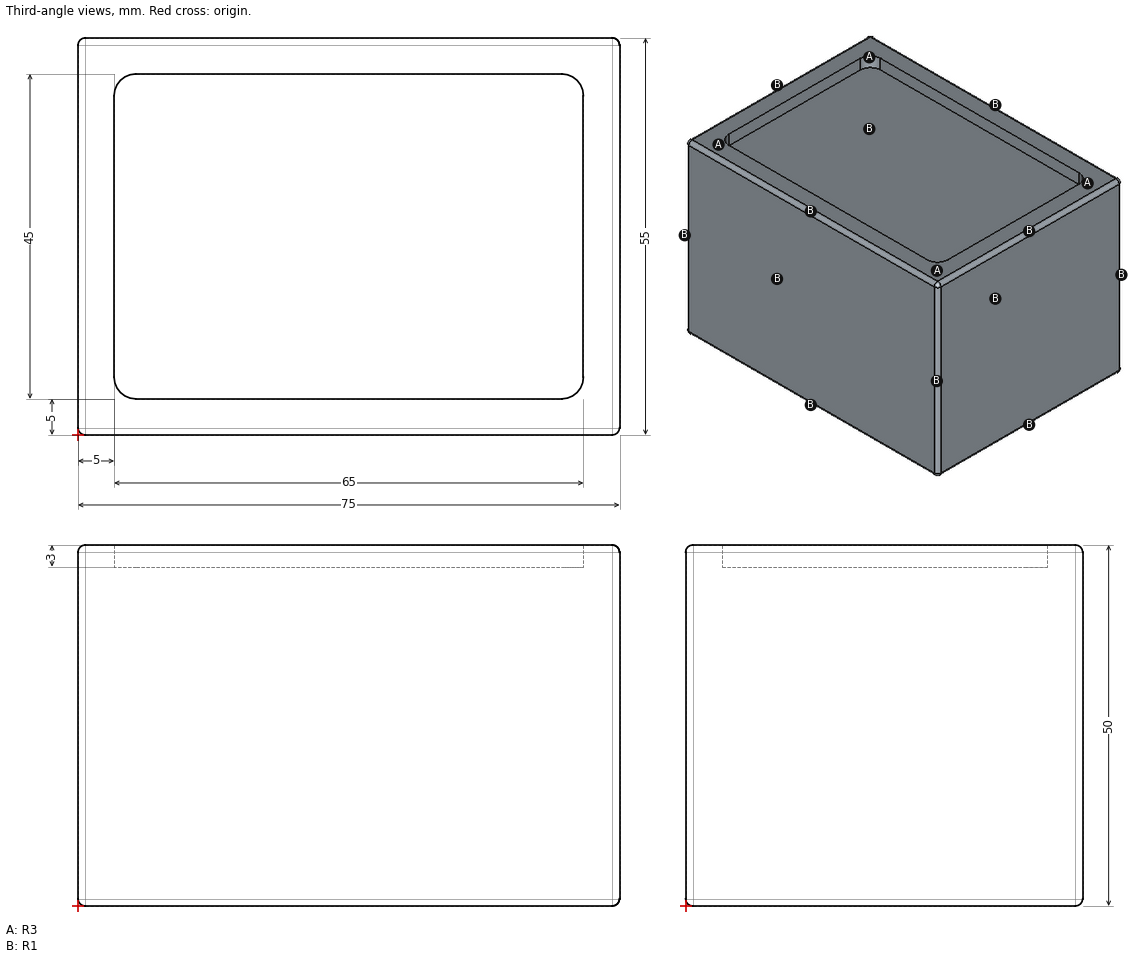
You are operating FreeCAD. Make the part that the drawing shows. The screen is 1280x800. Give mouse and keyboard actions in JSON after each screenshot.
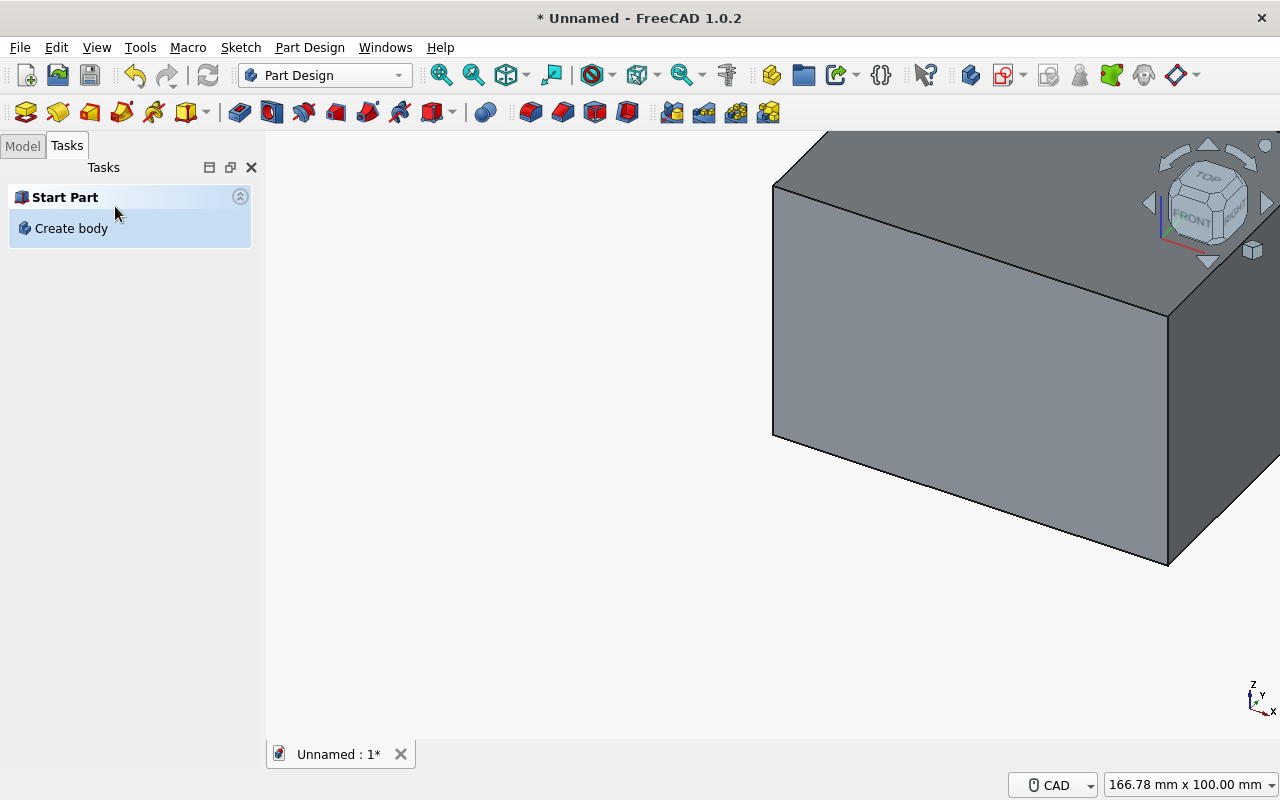
{"action": "left_click", "coordinate": [442, 76]}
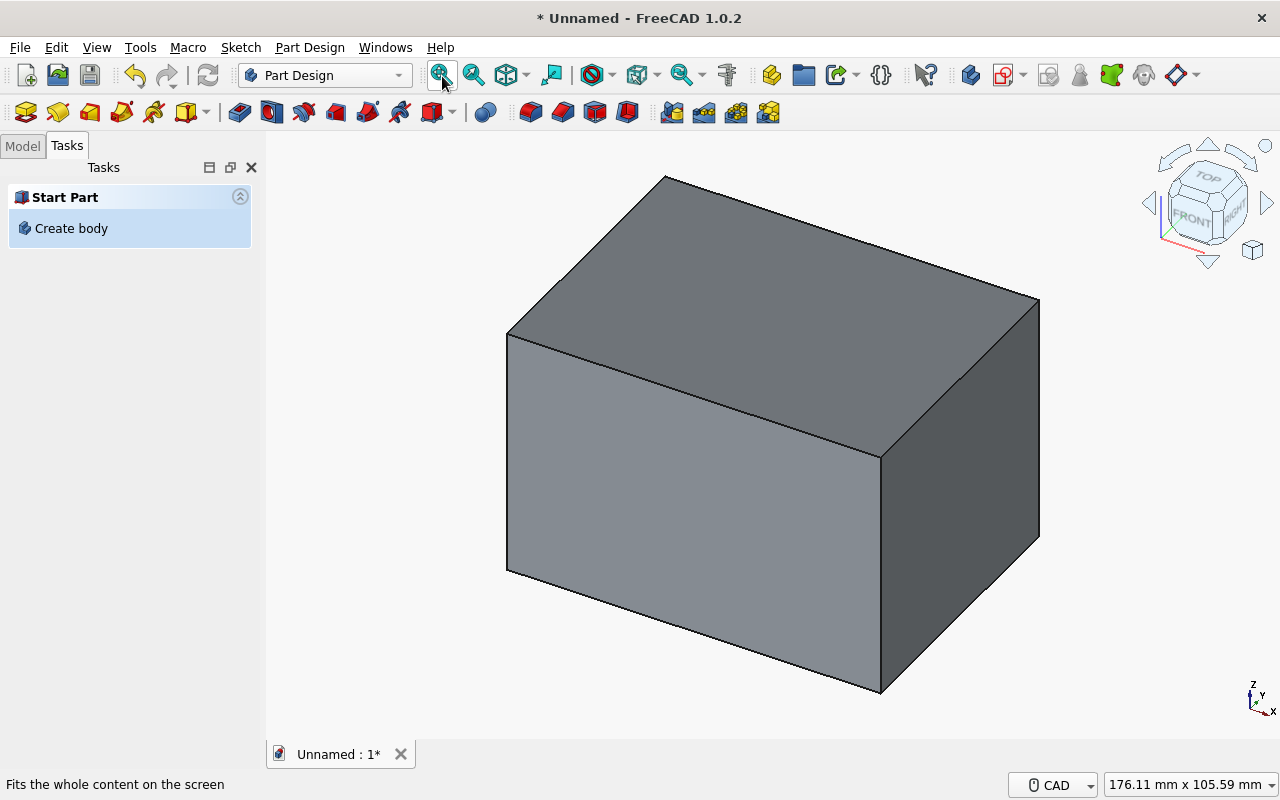
{"action": "left_click", "coordinate": [773, 316]}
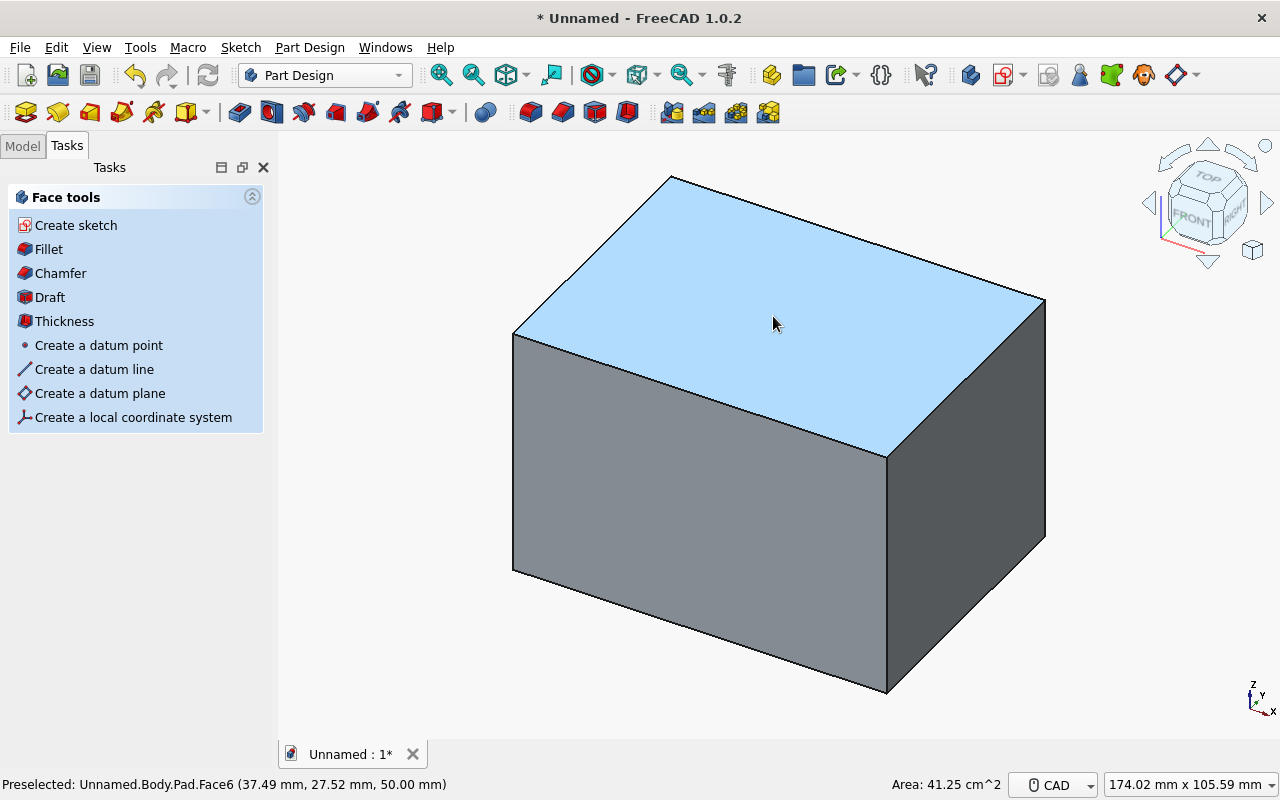
{"action": "left_click", "coordinate": [1004, 76]}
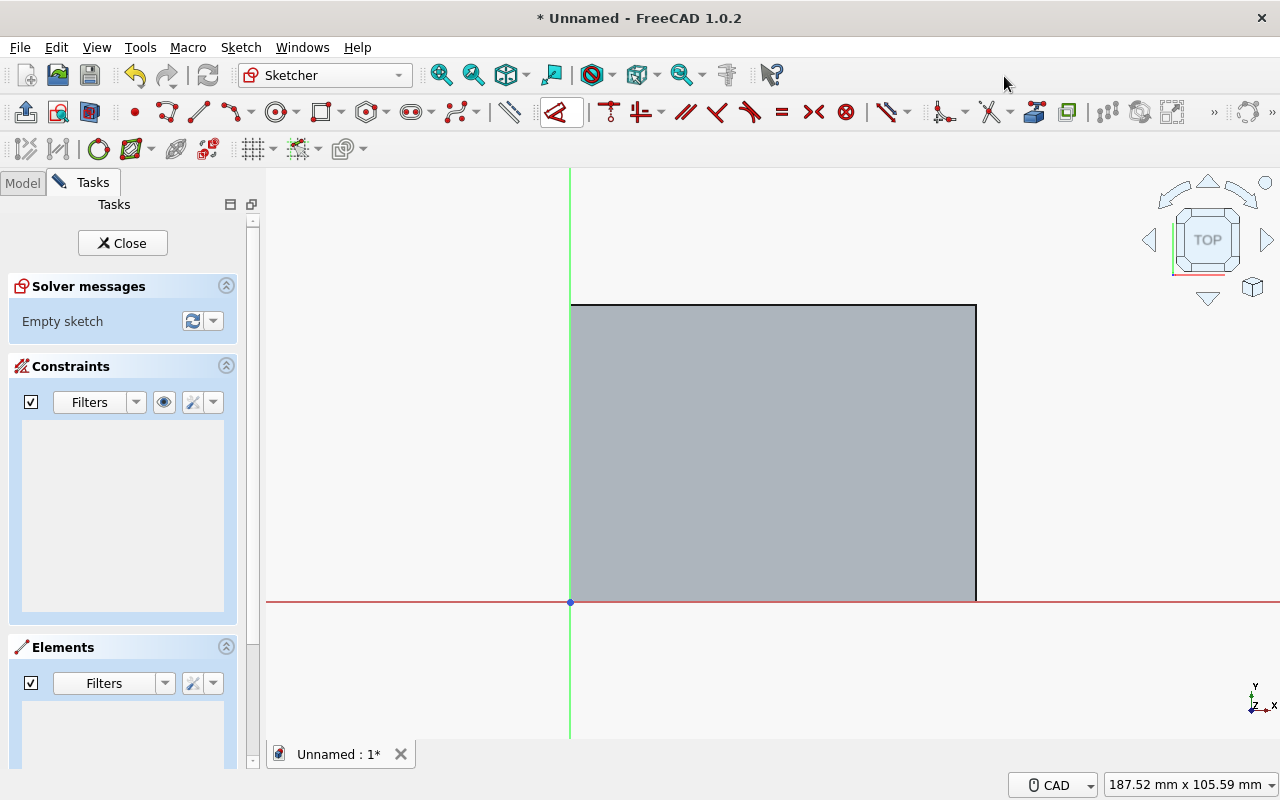
{"action": "left_click", "coordinate": [322, 112]}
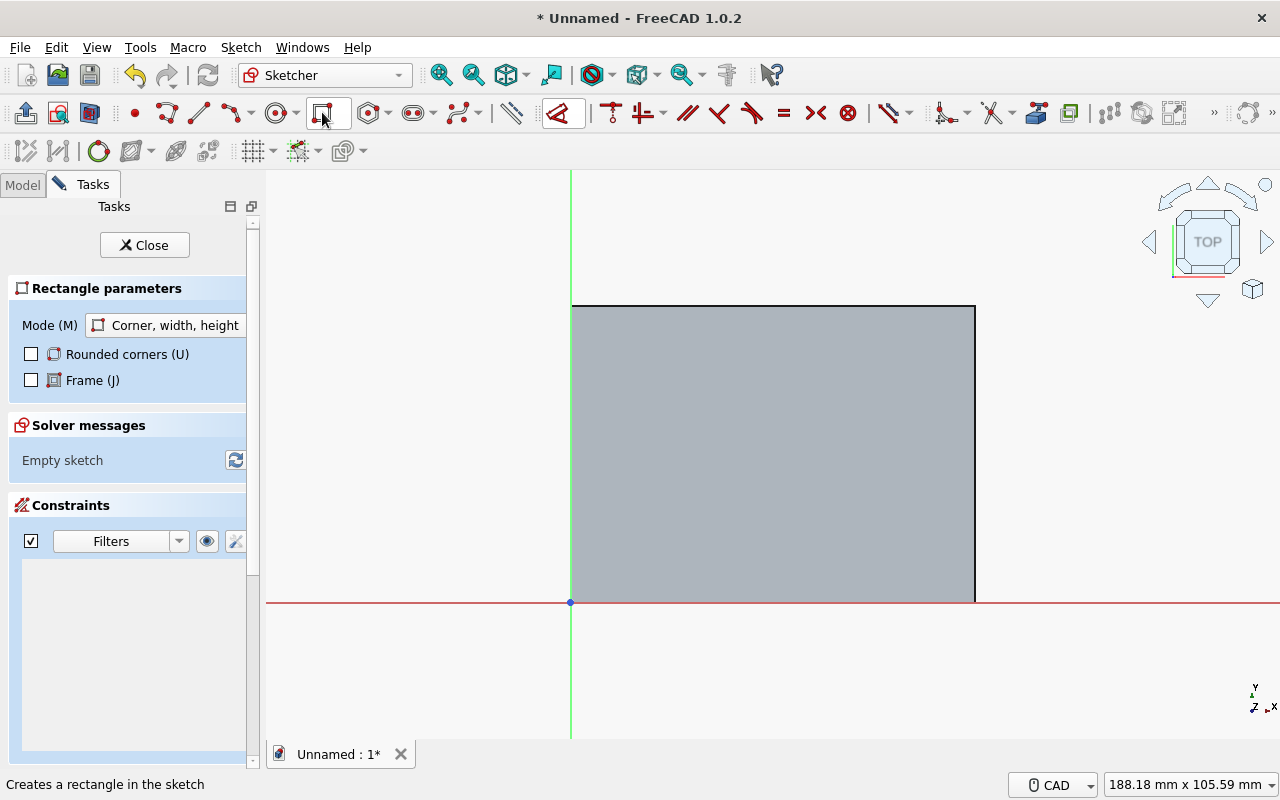
{"action": "left_click", "coordinate": [598, 333]}
{"action": "left_click", "coordinate": [948, 576]}
{"action": "key", "text": "Escape"}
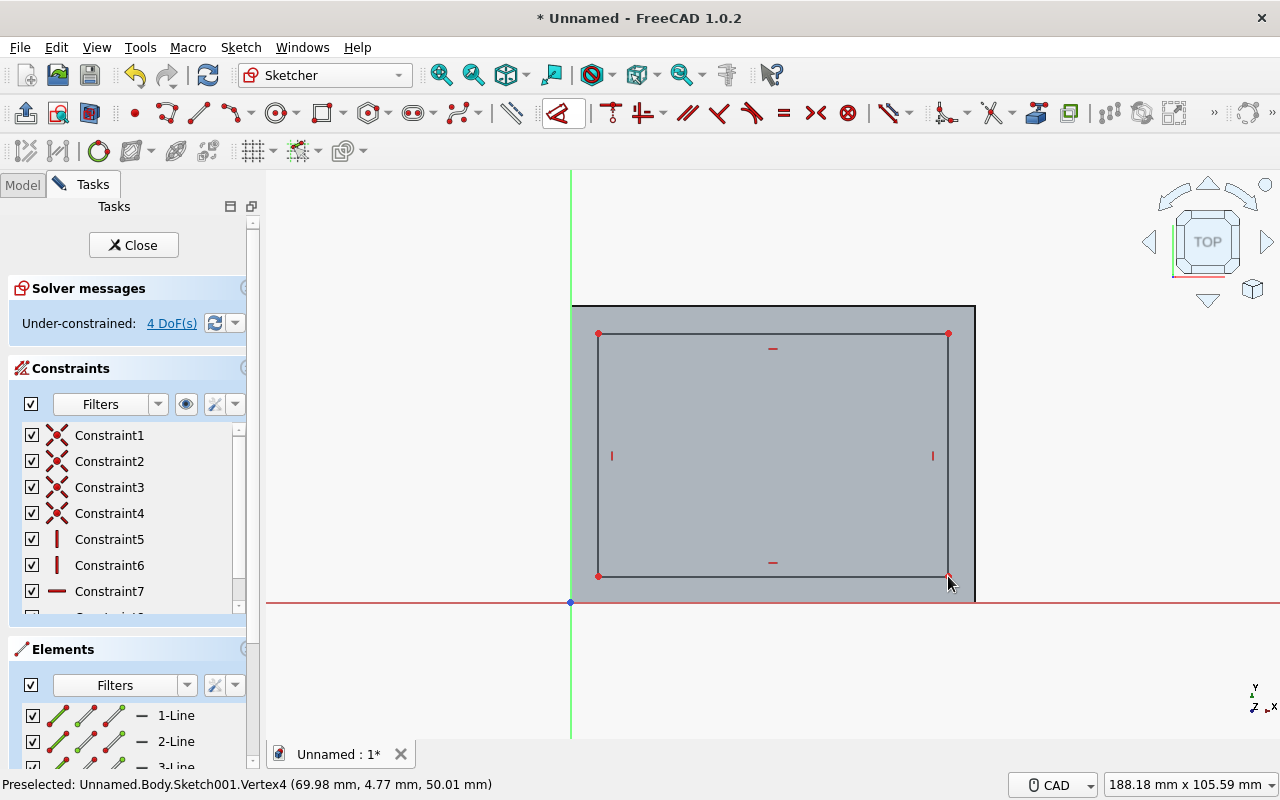
{"action": "left_click", "coordinate": [598, 407]}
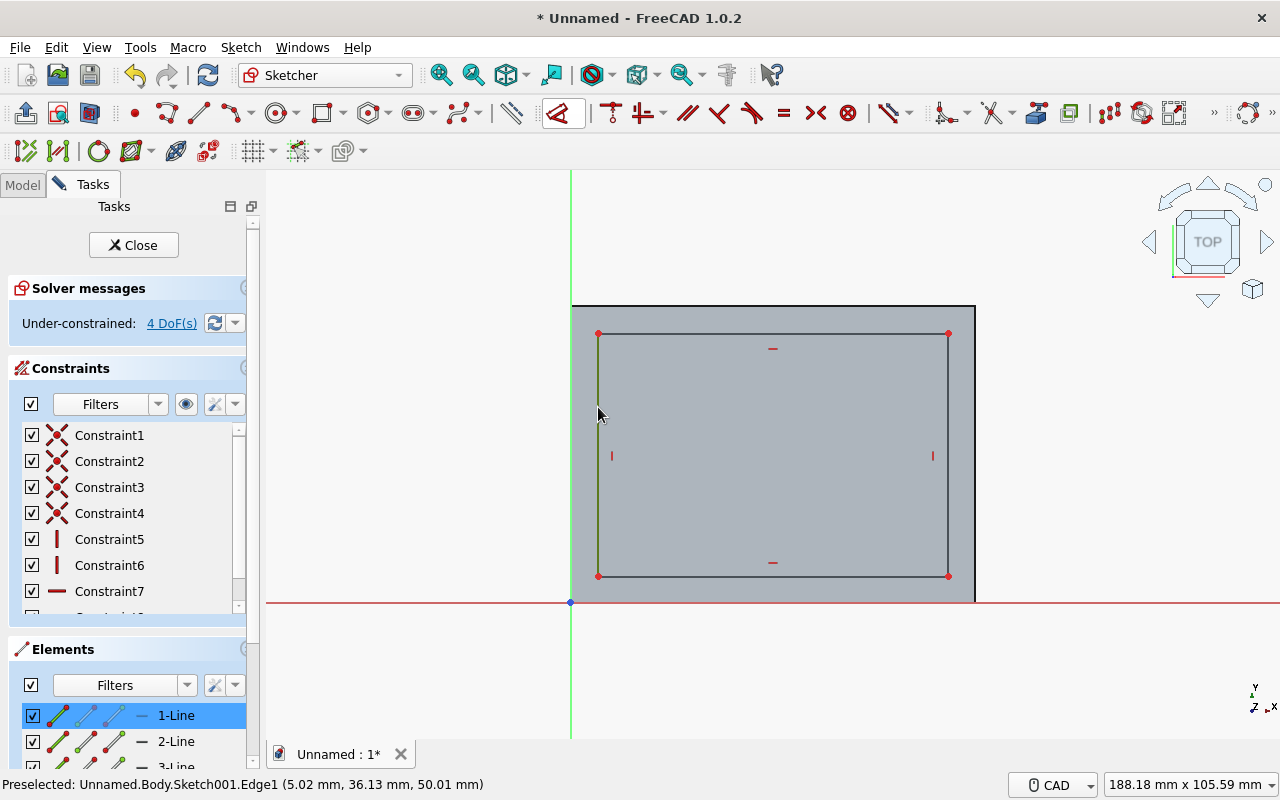
{"action": "left_click", "coordinate": [580, 114]}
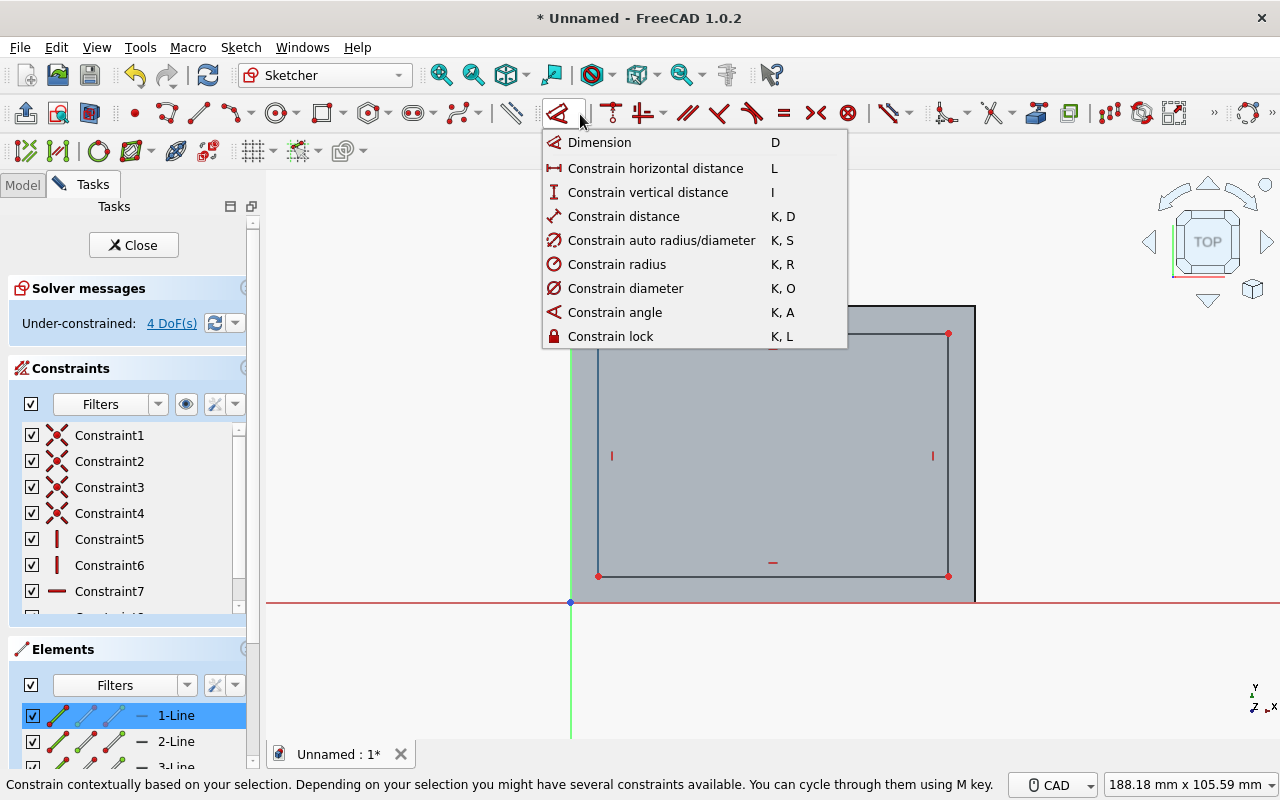
{"action": "left_click", "coordinate": [695, 192]}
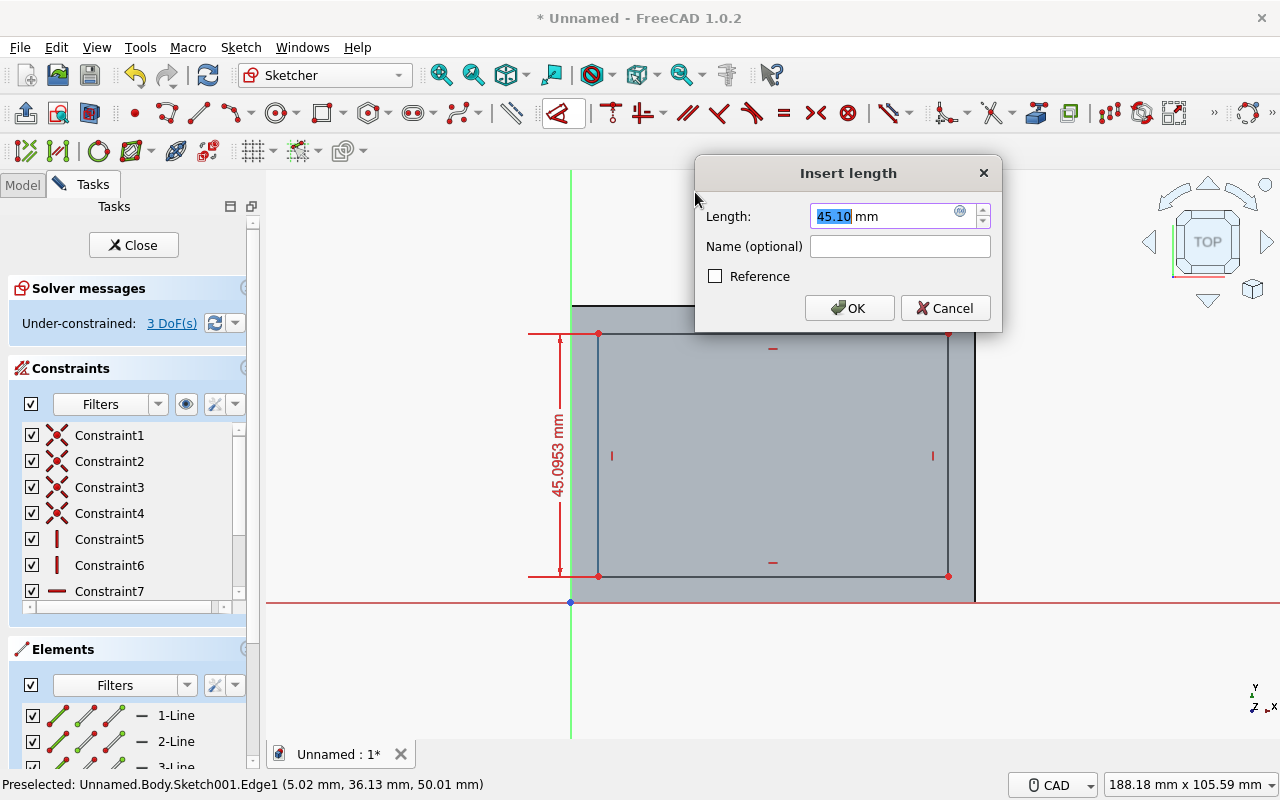
{"action": "type", "text": "45"}
{"action": "key", "text": "Return"}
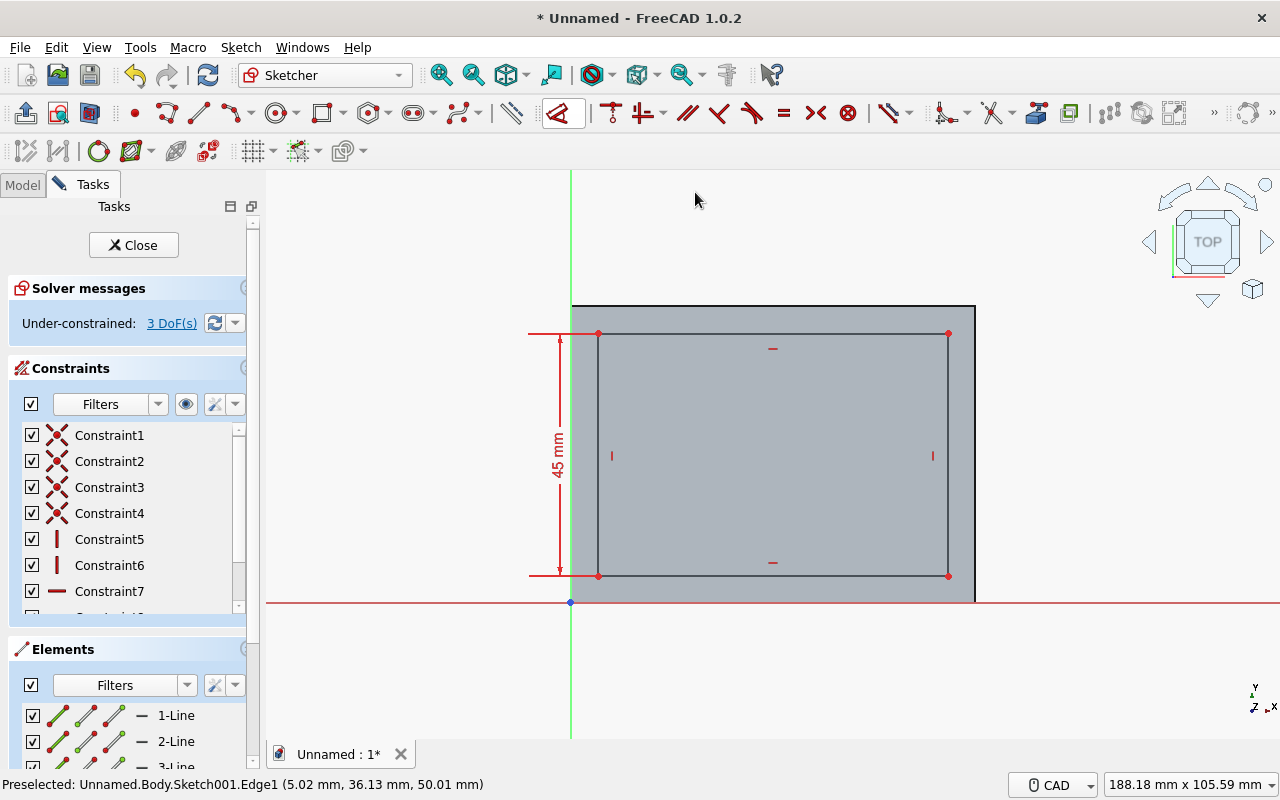
{"action": "left_click", "coordinate": [703, 576]}